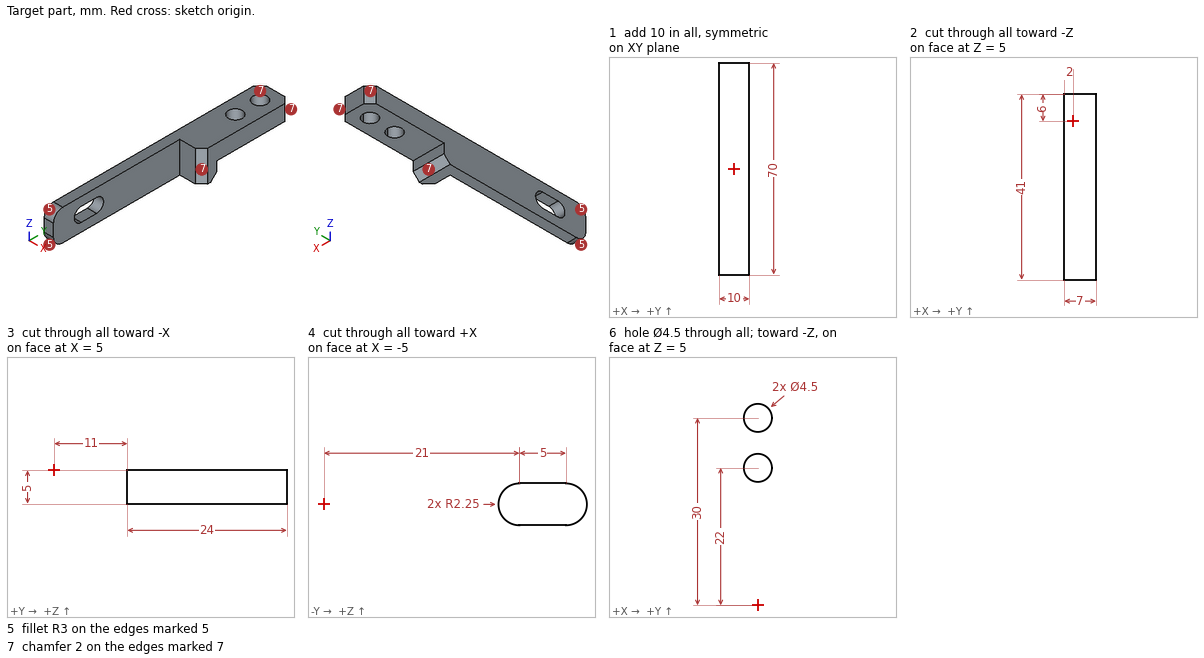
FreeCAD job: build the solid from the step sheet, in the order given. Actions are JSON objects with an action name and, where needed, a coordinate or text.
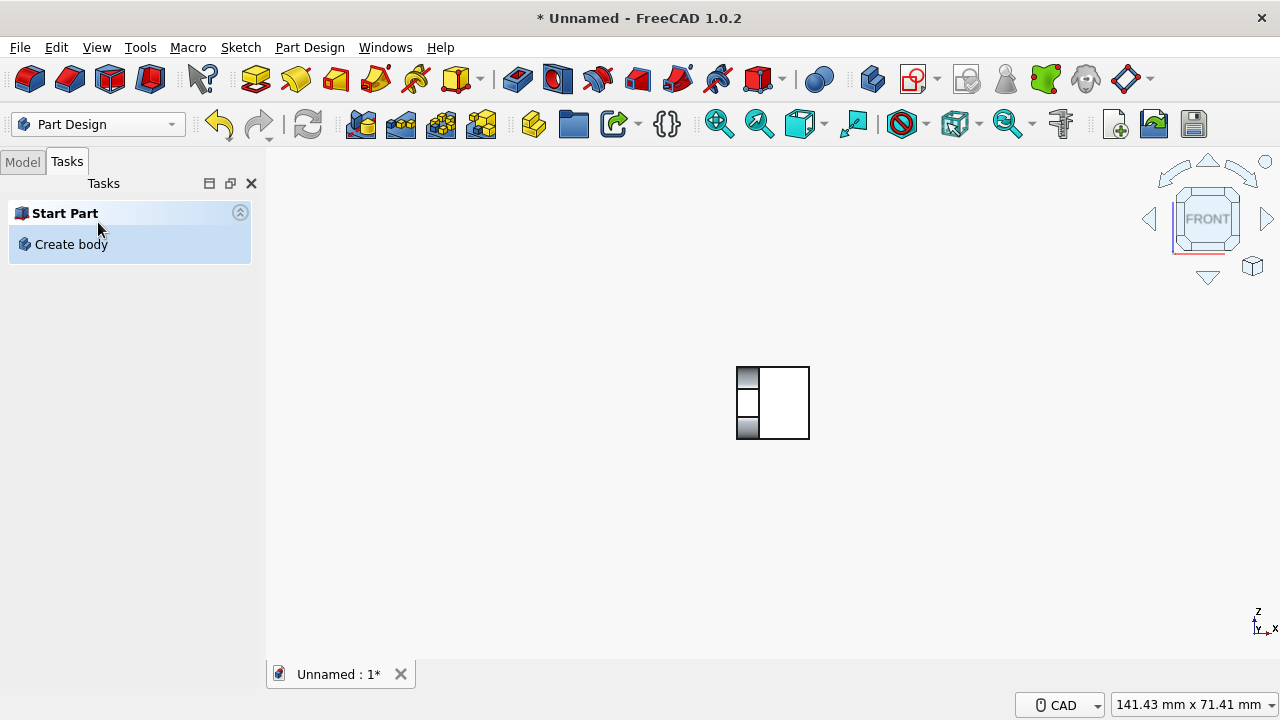
{"action": "key", "text": "v f"}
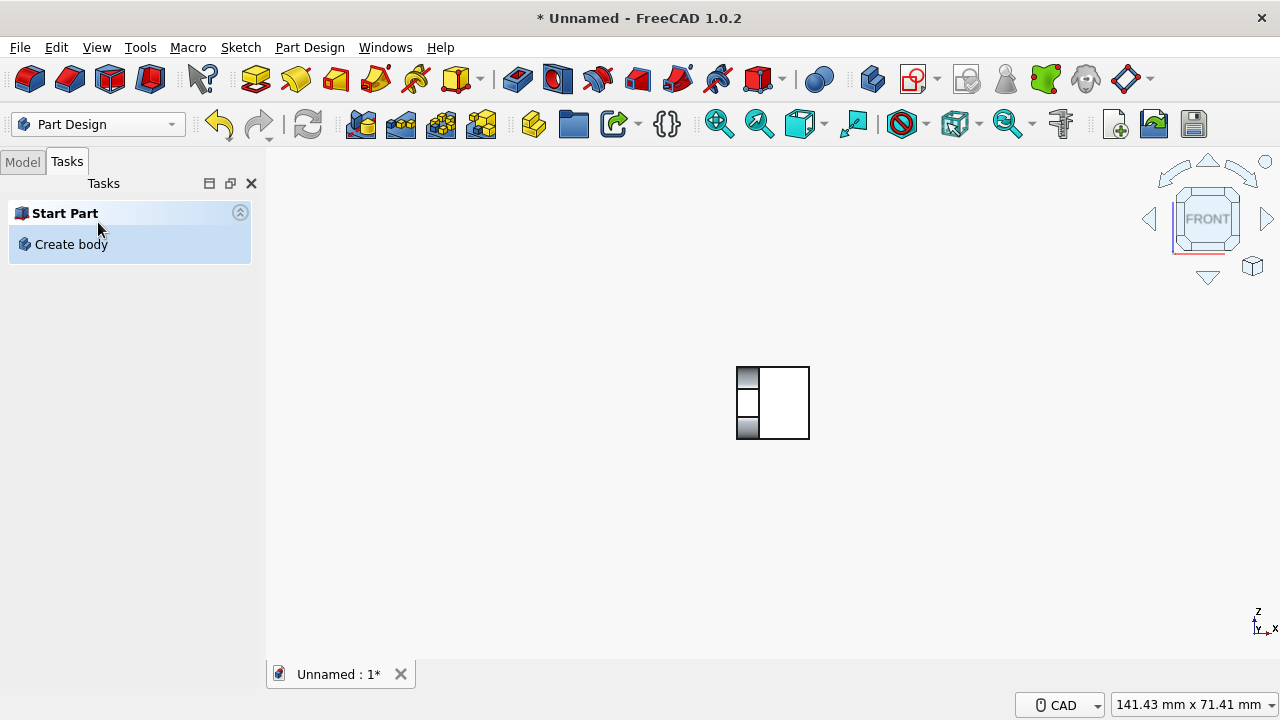
{"action": "key", "text": "0"}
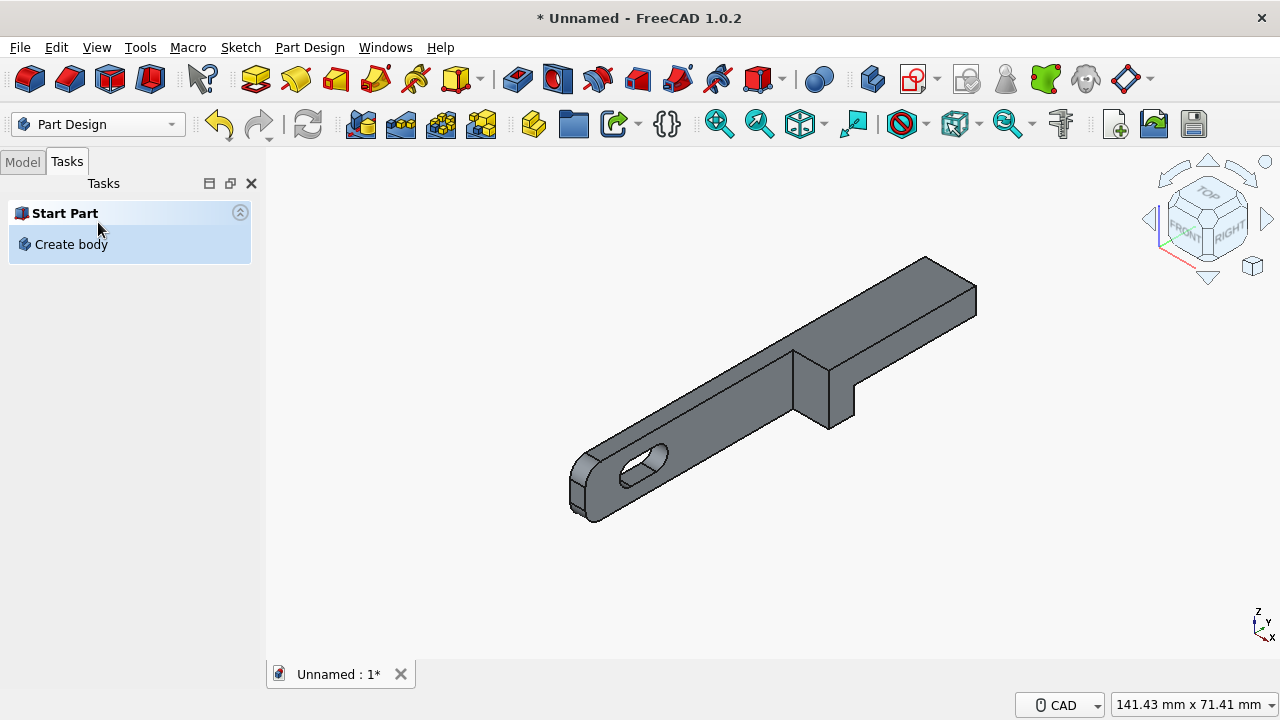
{"action": "left_click", "coordinate": [878, 312]}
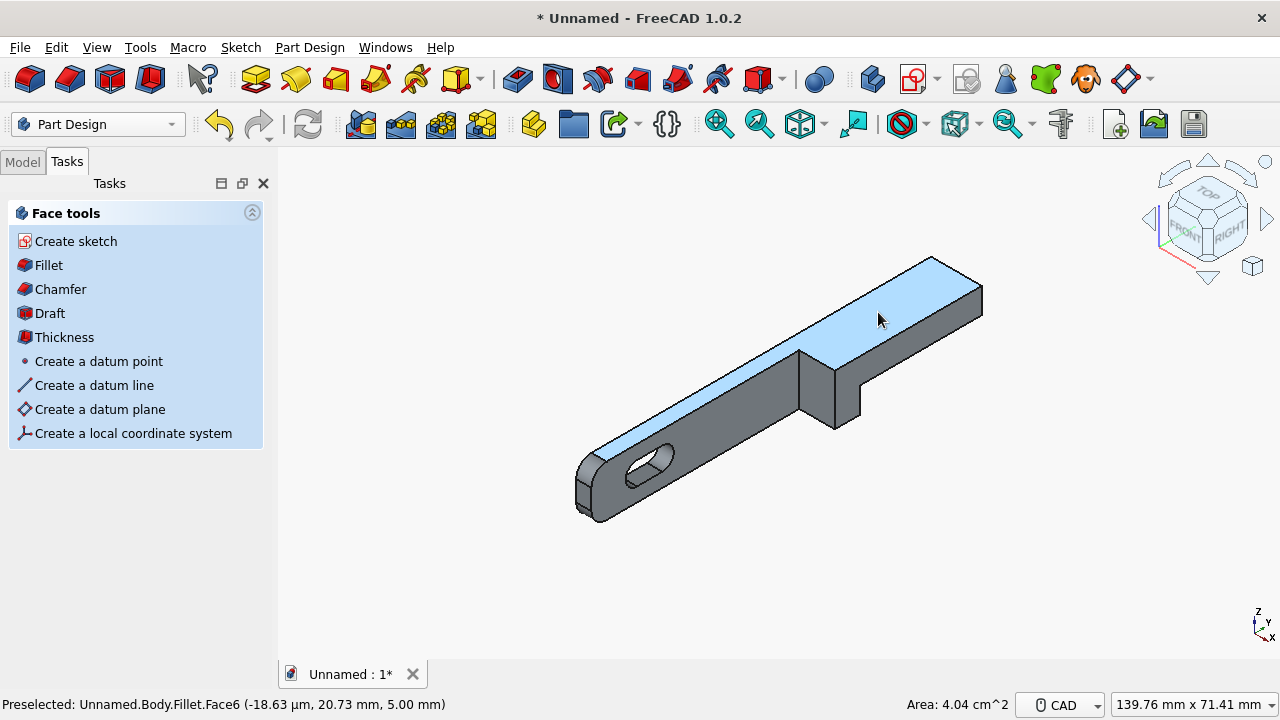
{"action": "left_click", "coordinate": [914, 80]}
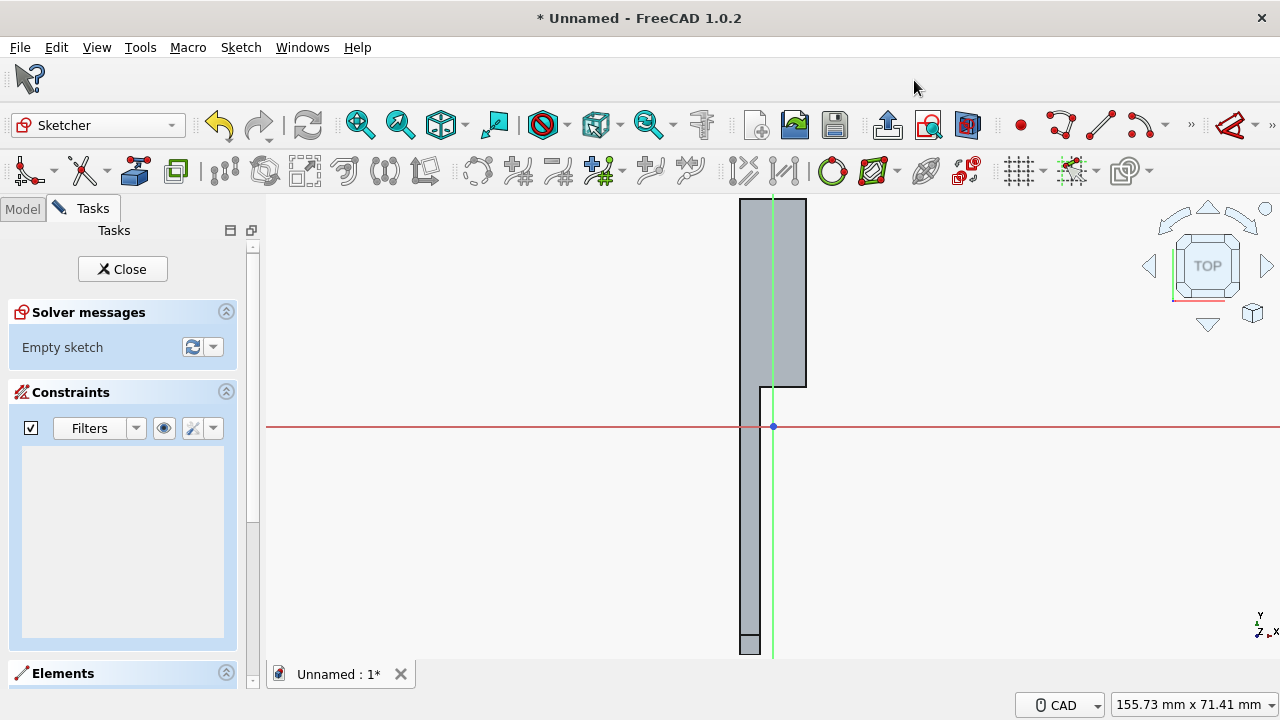
{"action": "scroll", "coordinate": [704, 426], "scroll_direction": "down", "scroll_amount": 5}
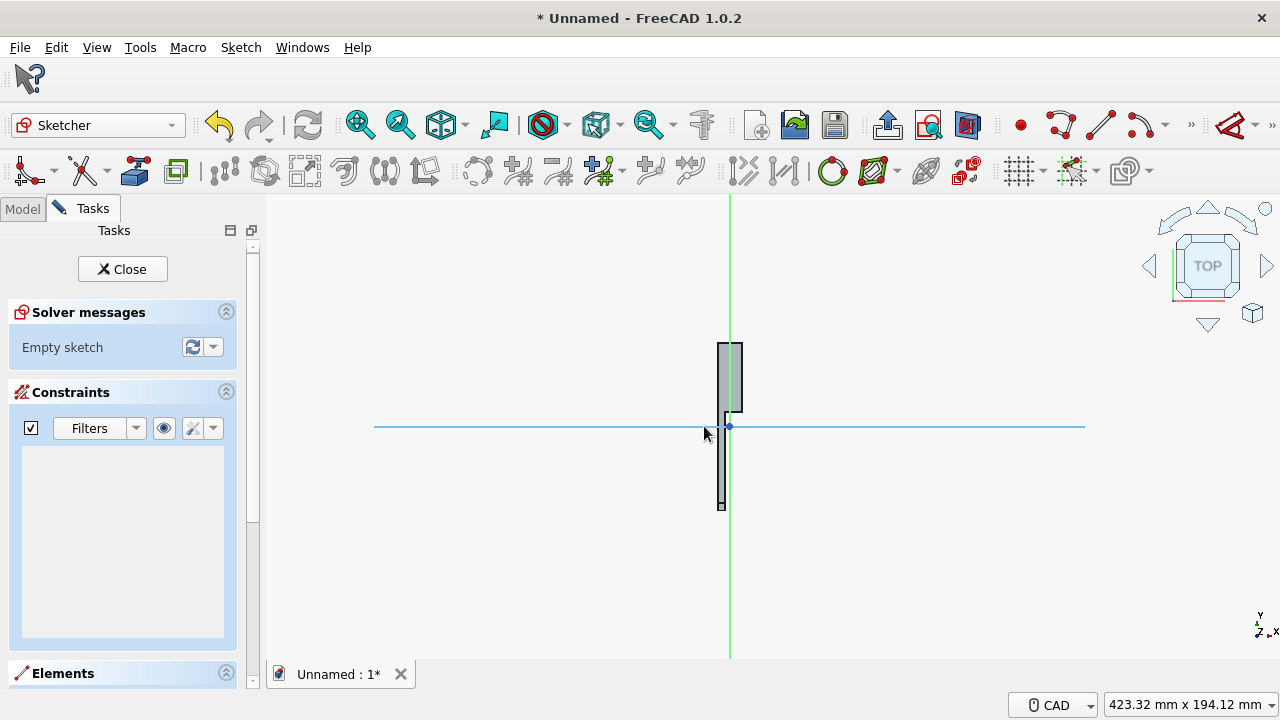
{"action": "scroll", "coordinate": [733, 356], "scroll_direction": "up", "scroll_amount": 11}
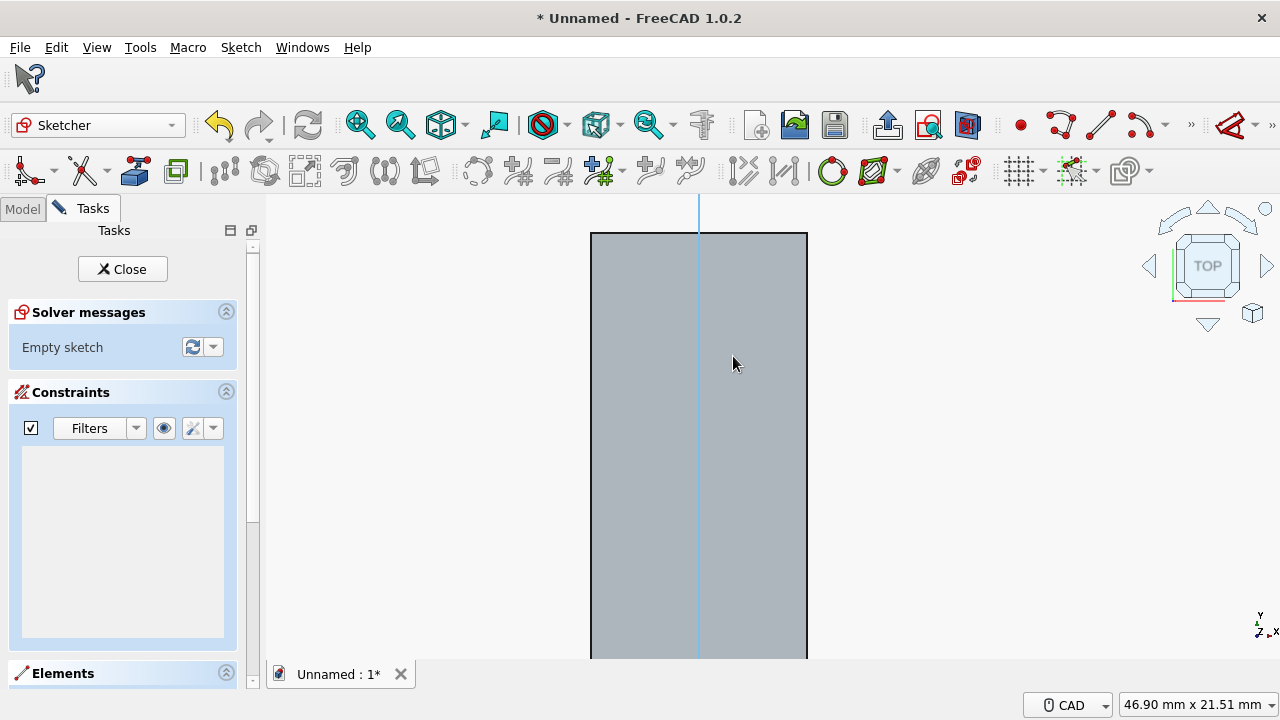
{"action": "key", "text": "g c"}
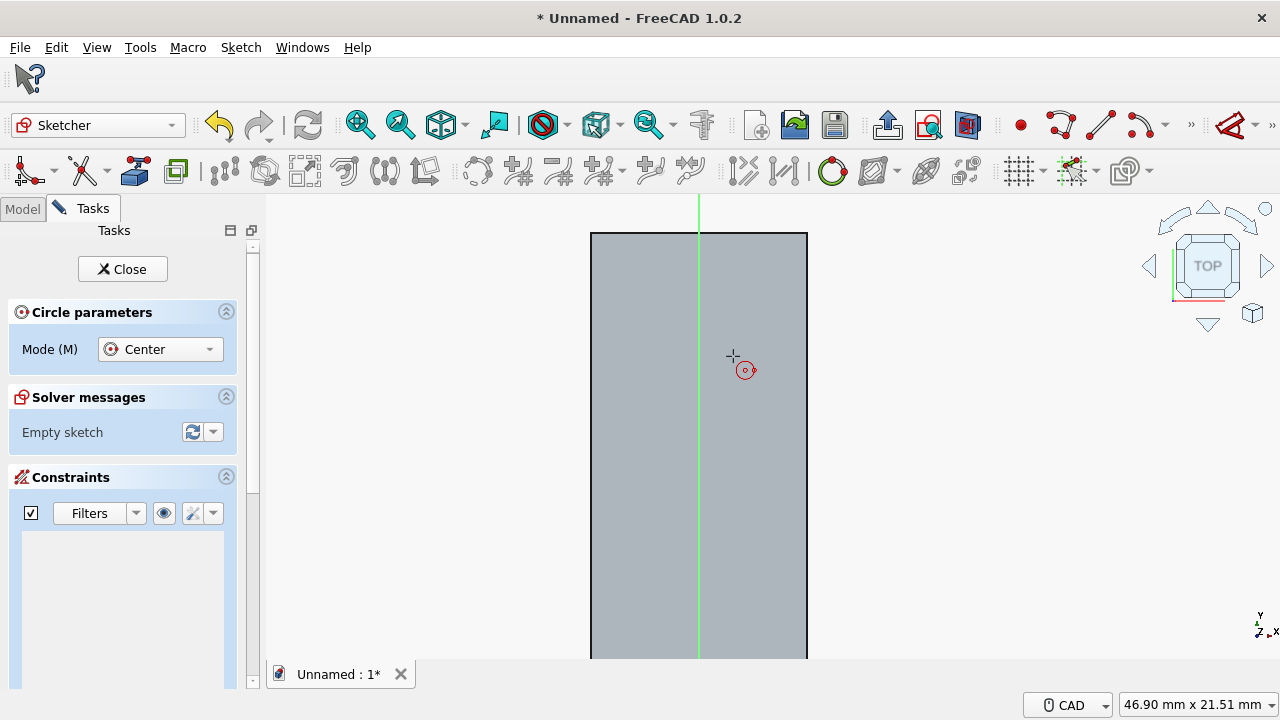
{"action": "left_click", "coordinate": [699, 341]}
{"action": "left_click", "coordinate": [734, 307]}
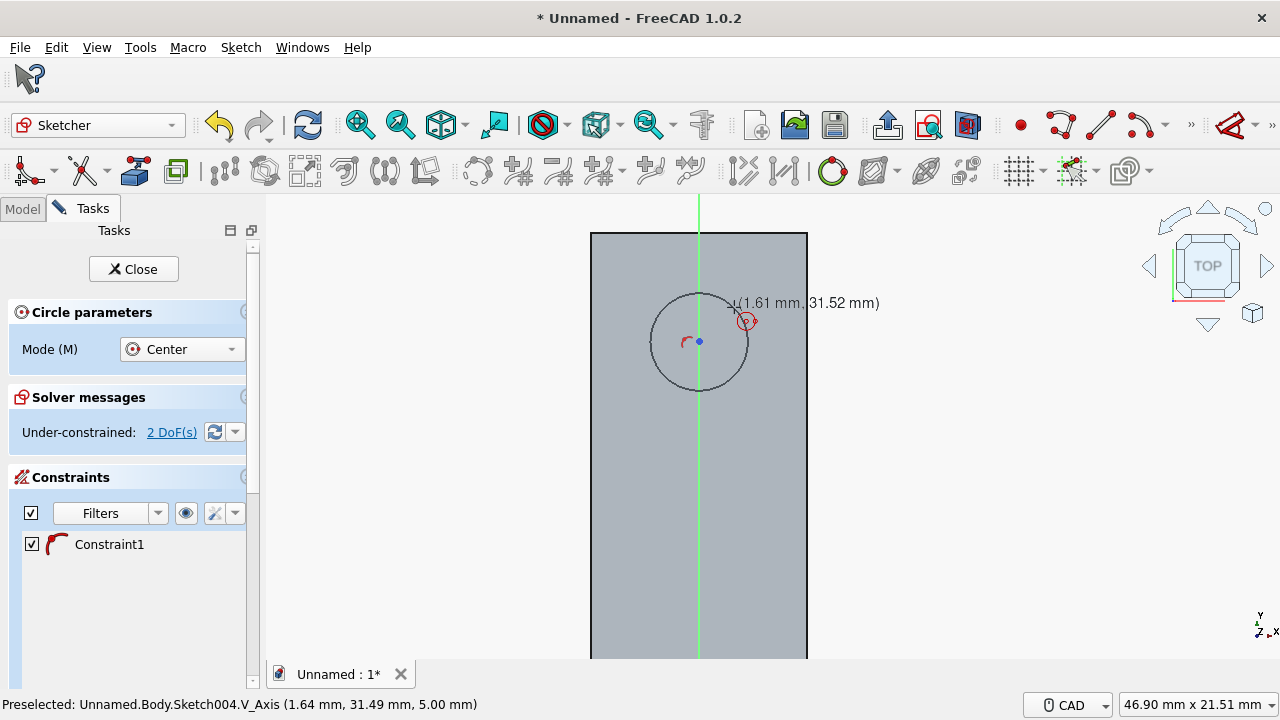
{"action": "left_click", "coordinate": [699, 514]}
{"action": "left_click", "coordinate": [734, 479]}
{"action": "key", "text": "Escape"}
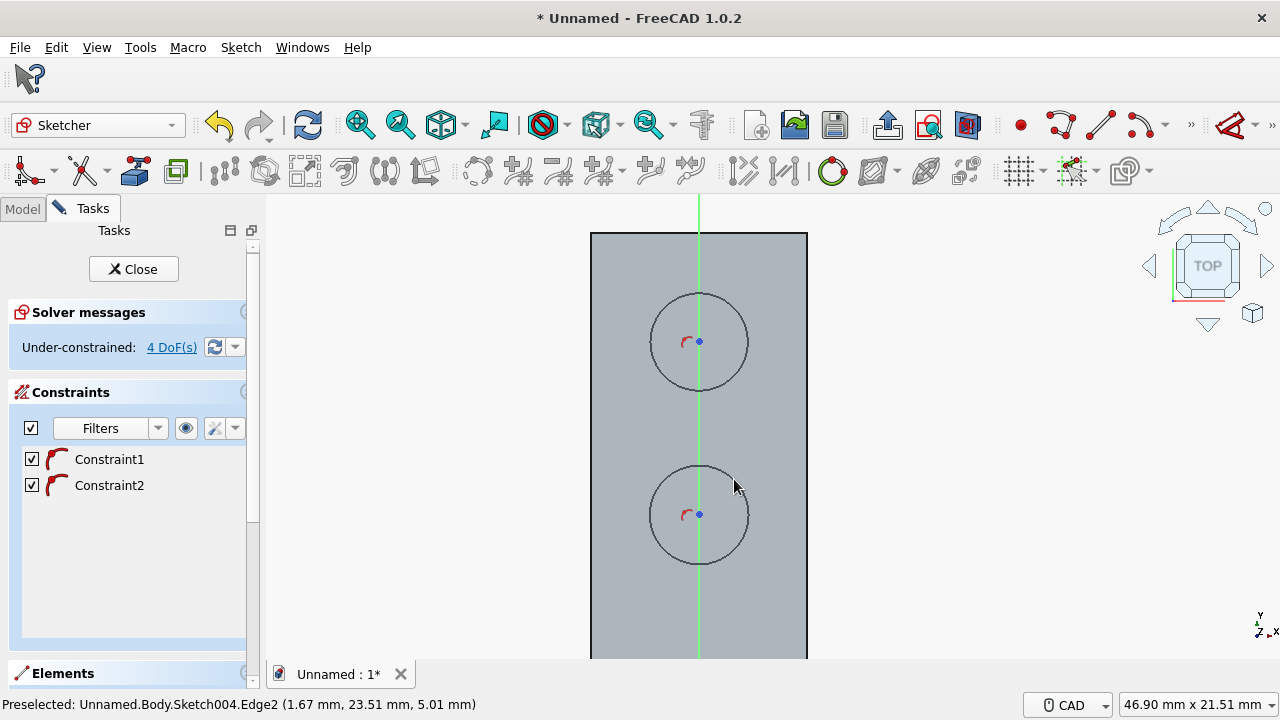
{"action": "left_click", "coordinate": [733, 307]}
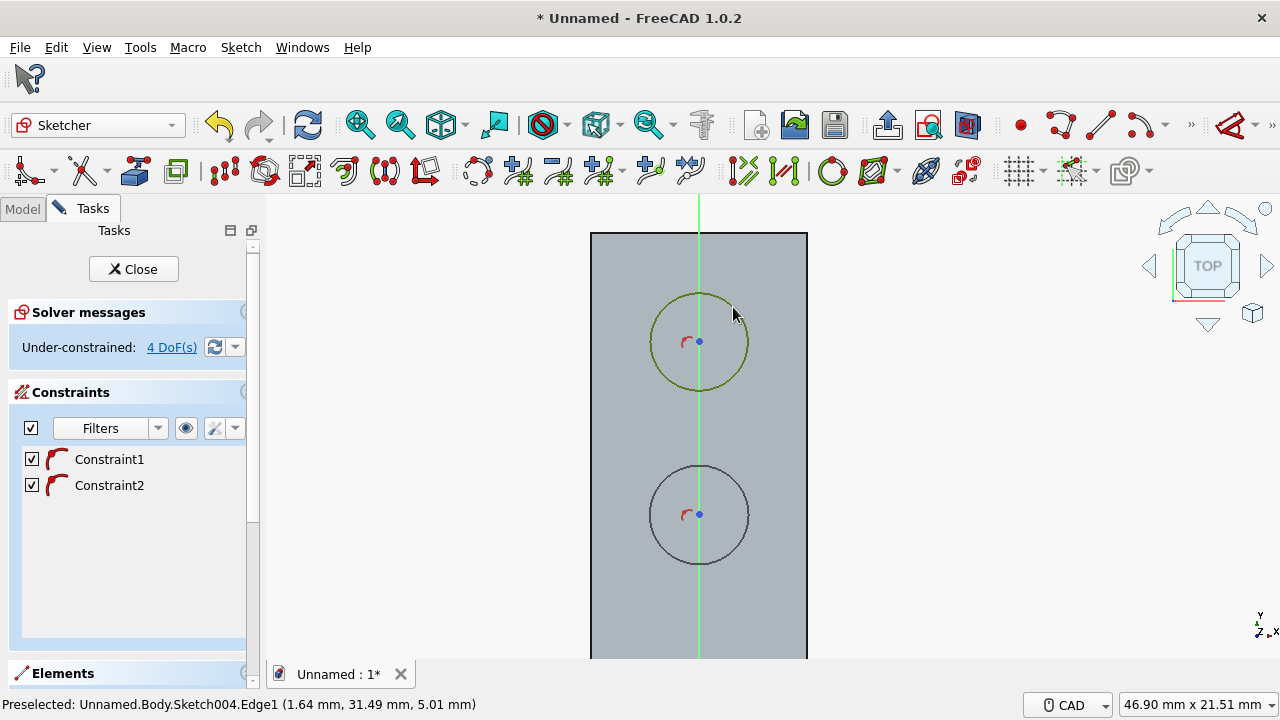
{"action": "left_click", "coordinate": [734, 480]}